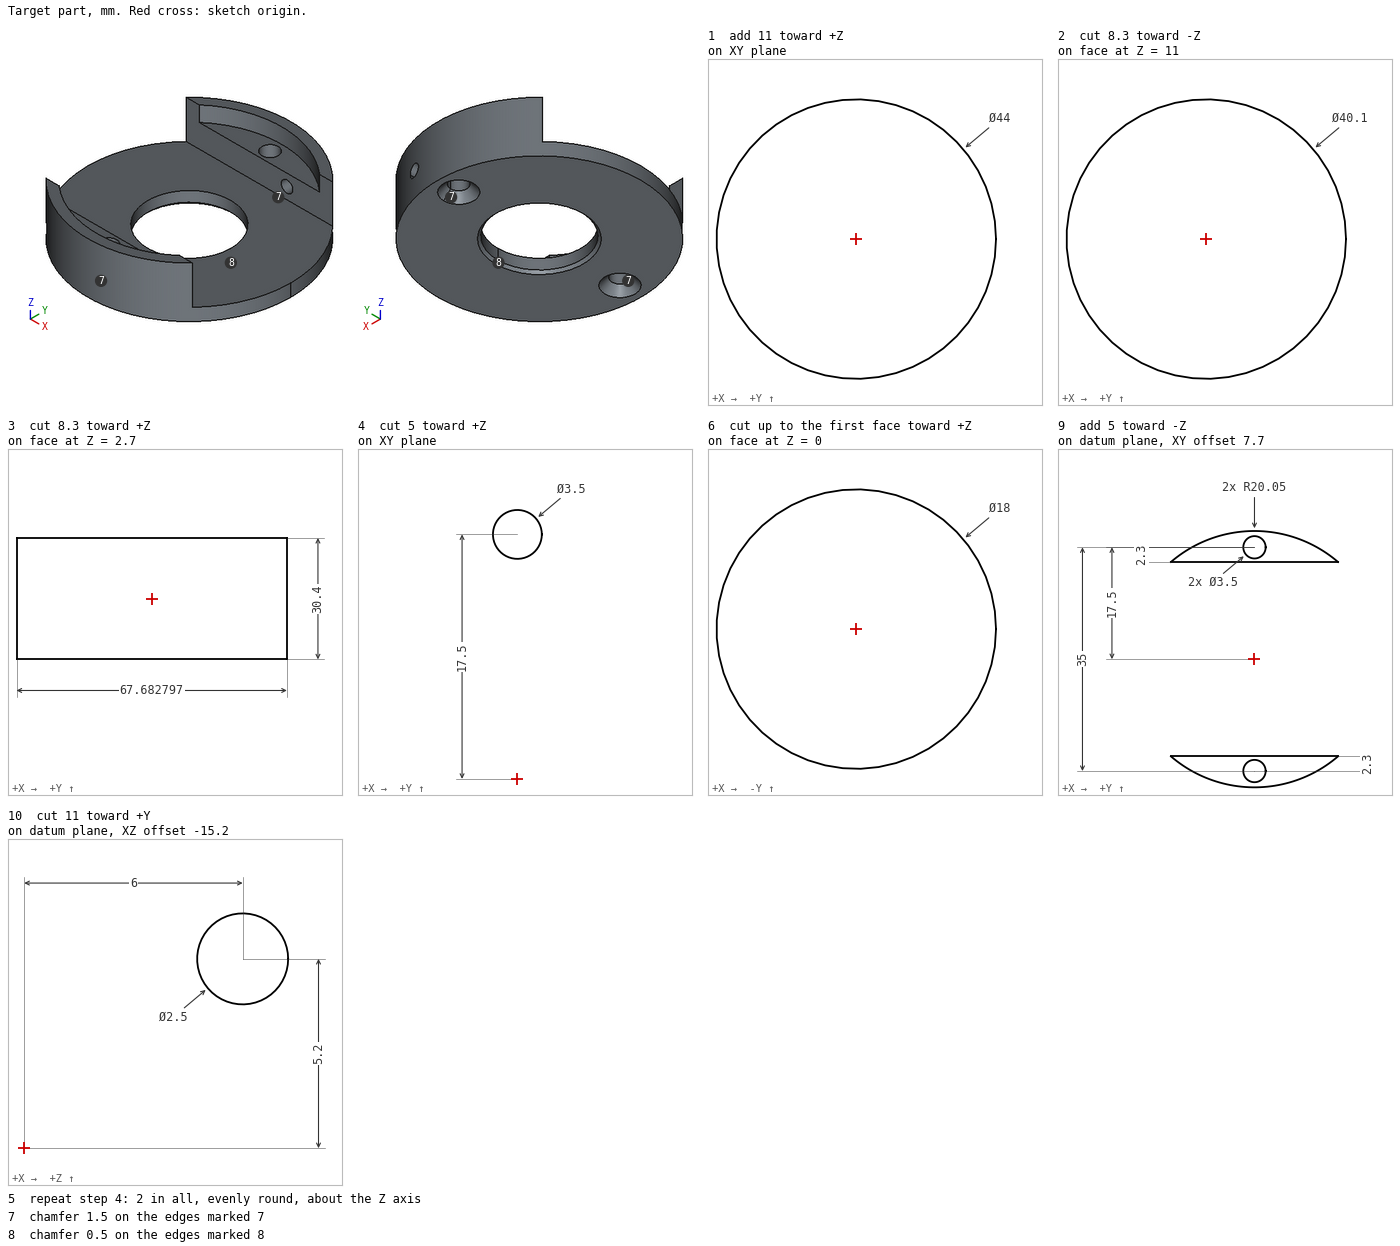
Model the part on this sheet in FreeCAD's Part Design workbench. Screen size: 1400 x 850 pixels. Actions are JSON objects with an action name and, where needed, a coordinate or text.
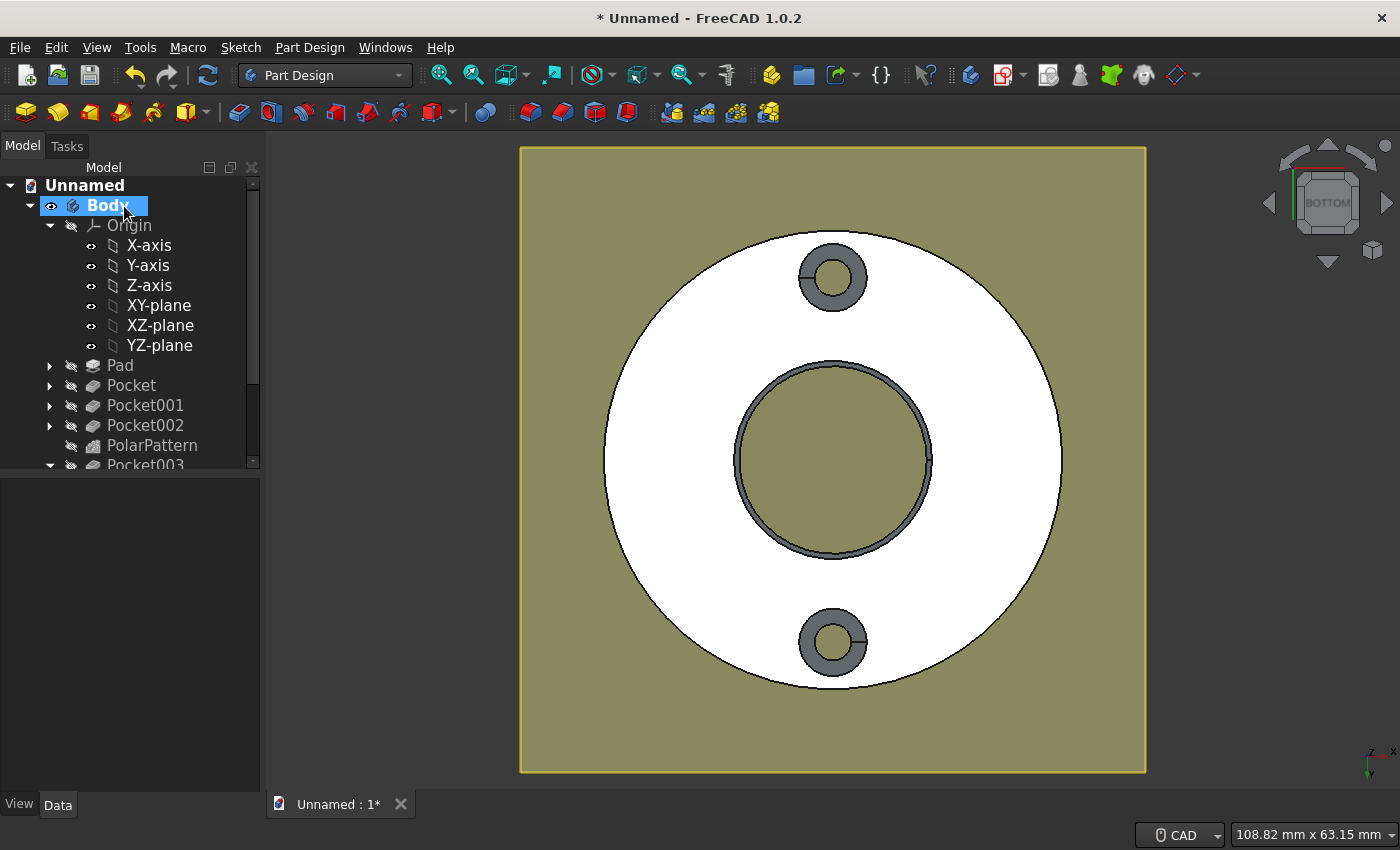
{"action": "scroll", "coordinate": [100, 321], "scroll_direction": "down", "scroll_amount": 3}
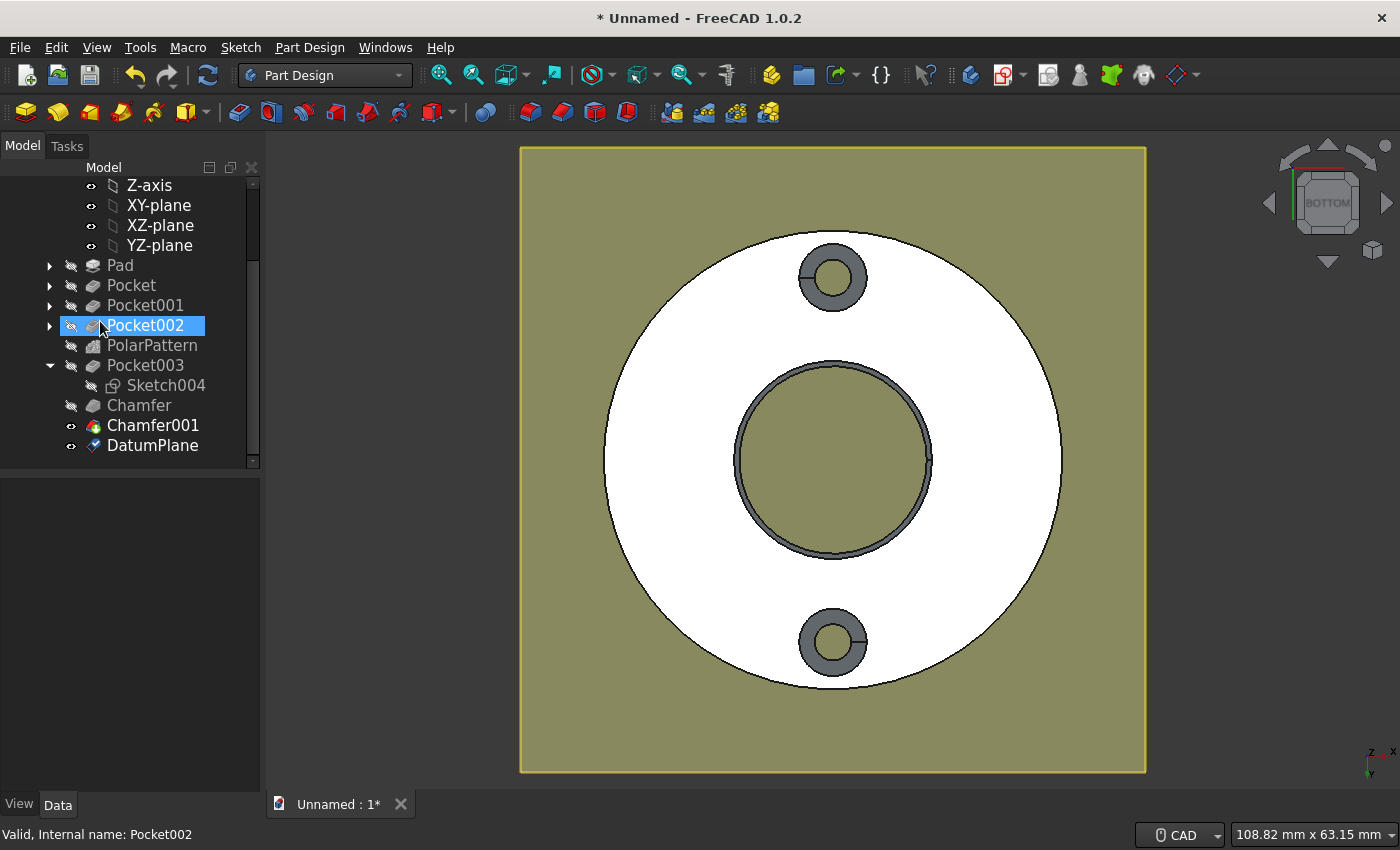
{"action": "left_click", "coordinate": [116, 446]}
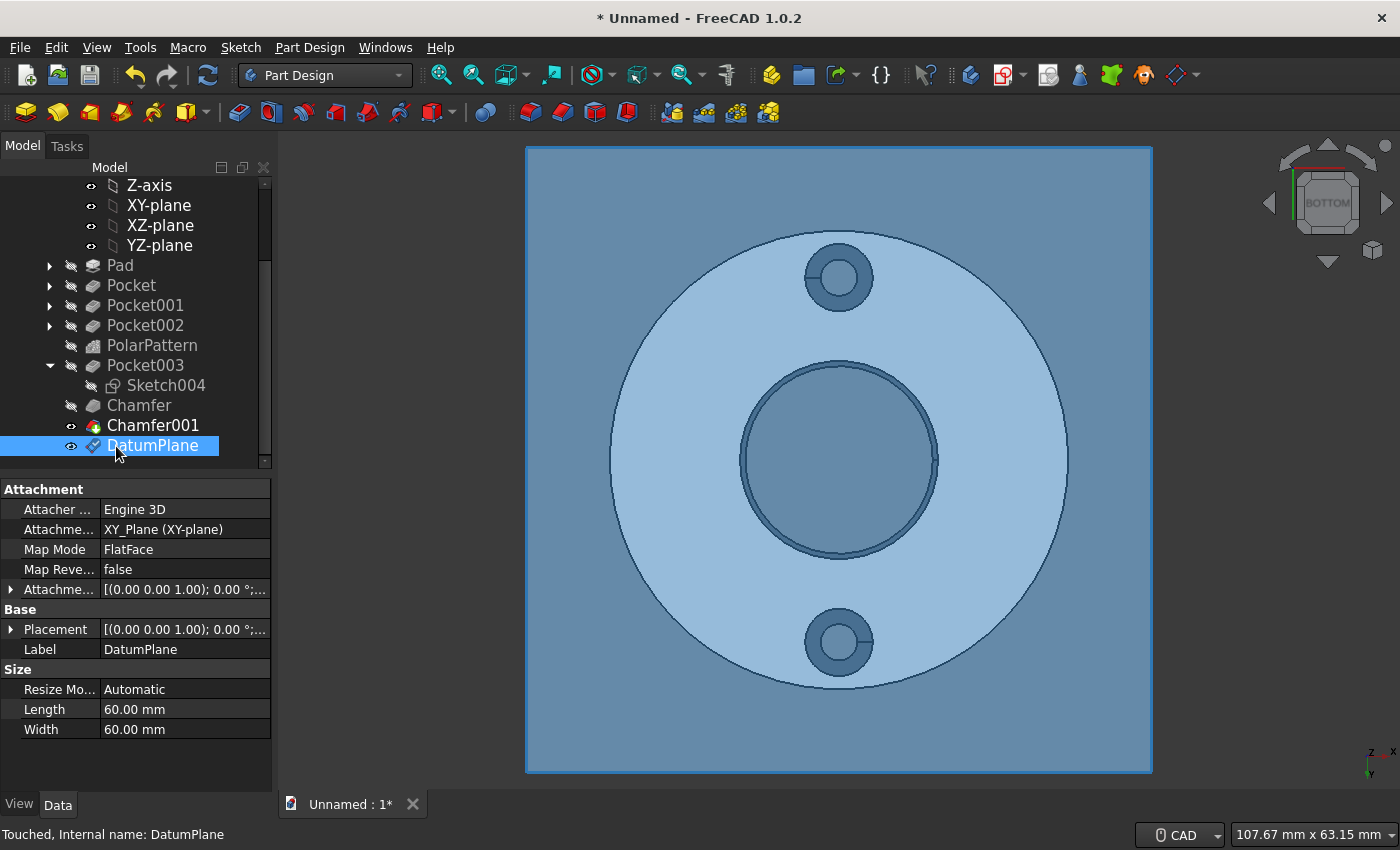
{"action": "left_click", "coordinate": [1004, 76]}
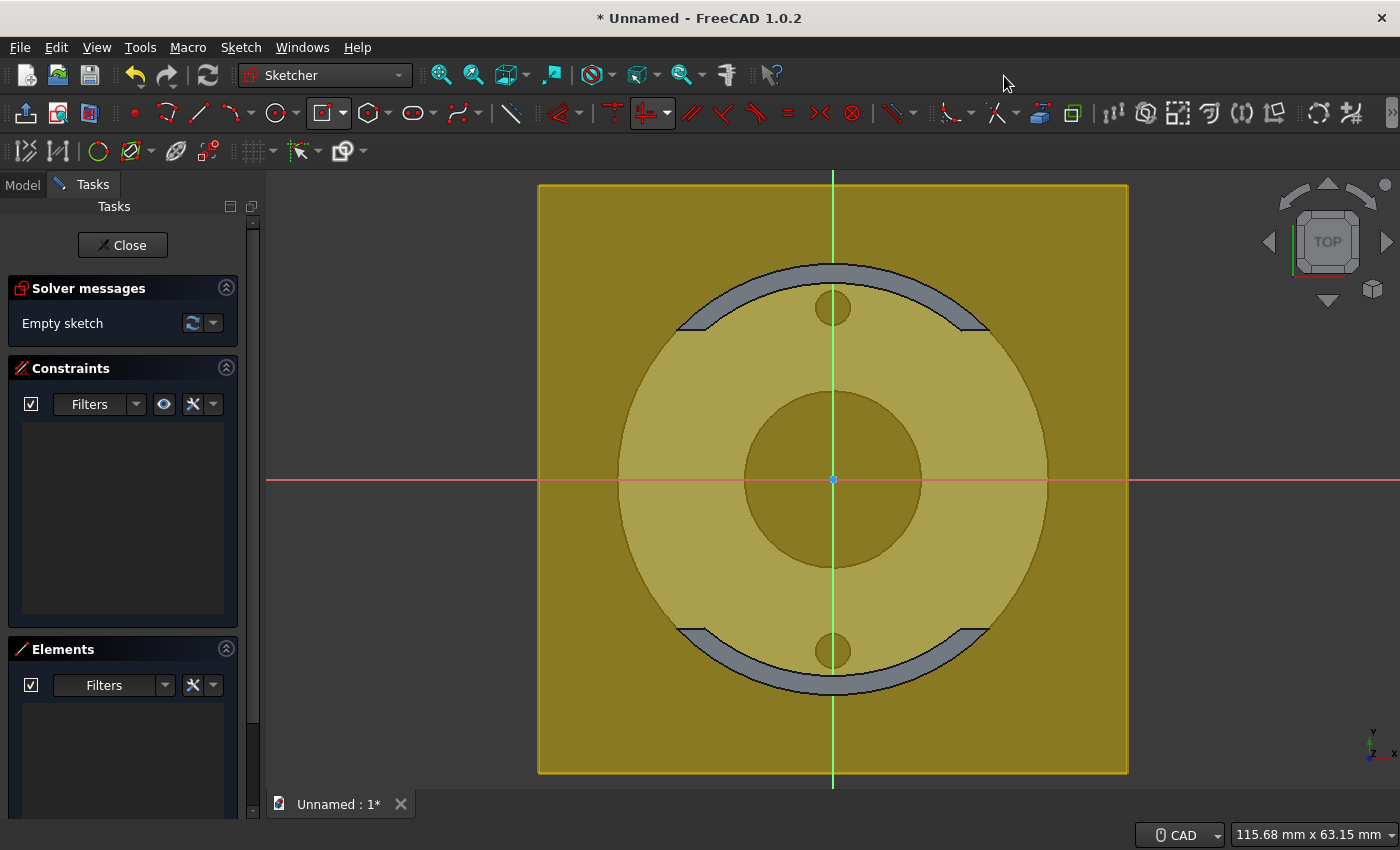
{"action": "left_click", "coordinate": [90, 114]}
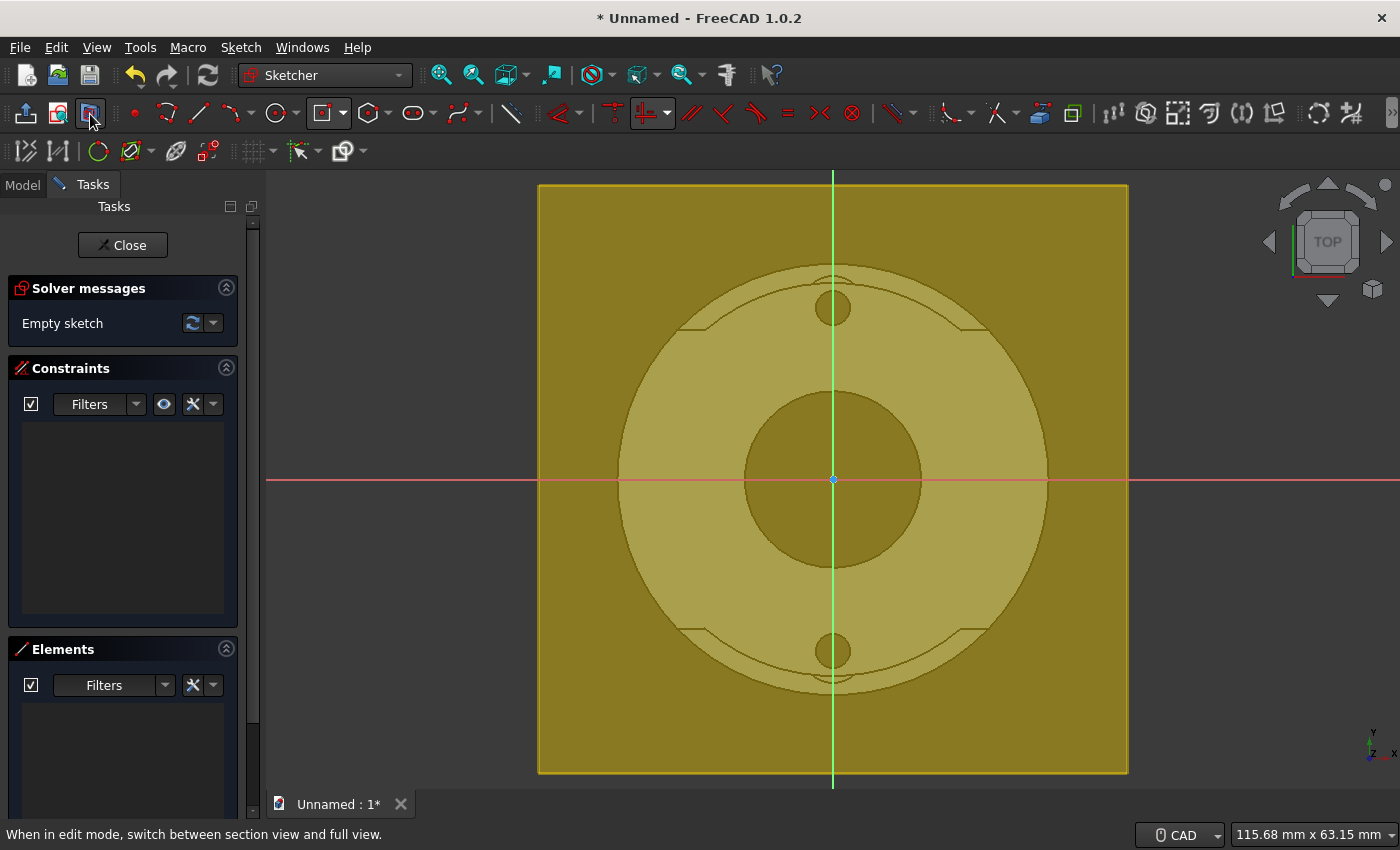
{"action": "key", "text": "g l"}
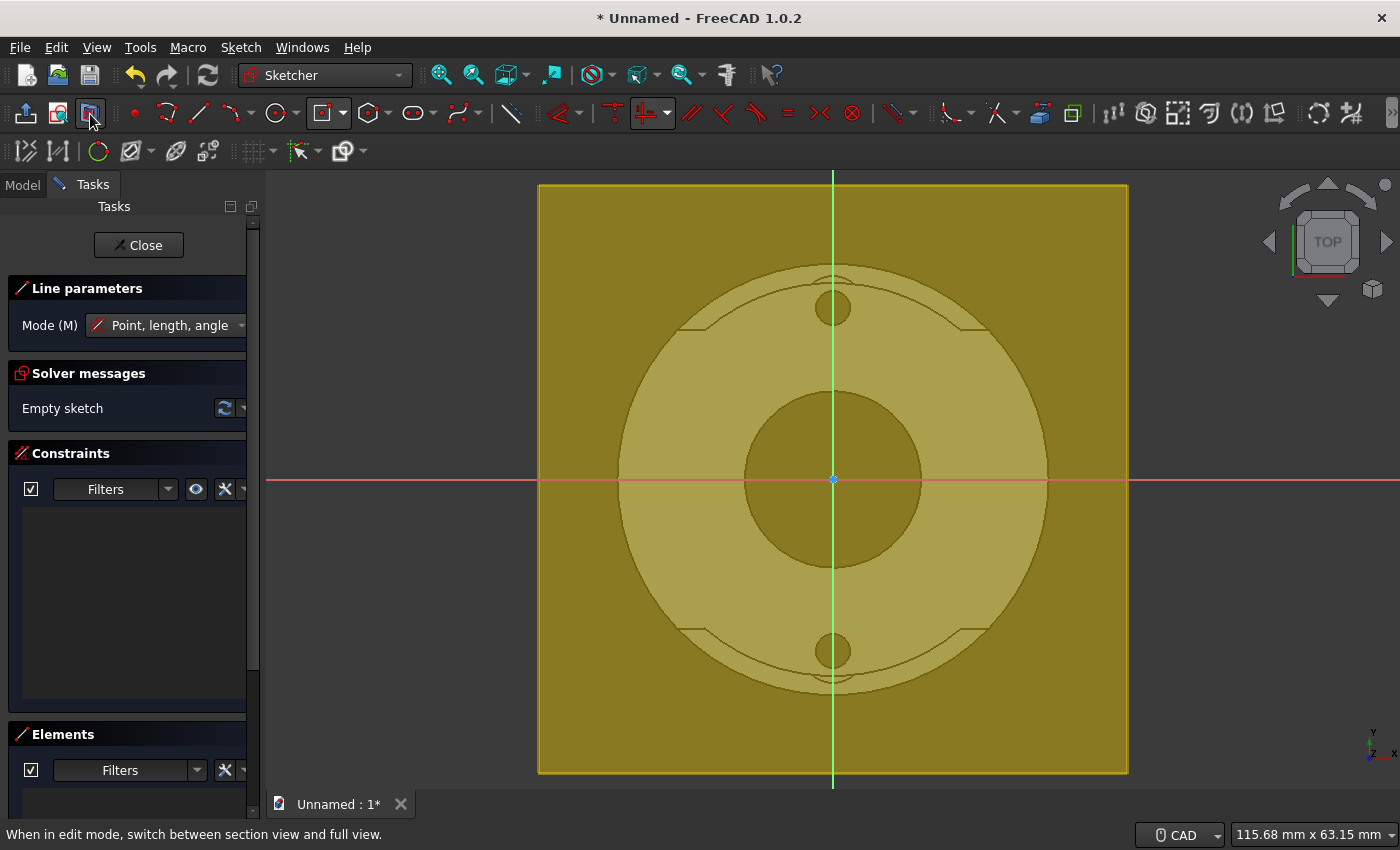
{"action": "left_click", "coordinate": [705, 330]}
{"action": "left_click", "coordinate": [961, 330]}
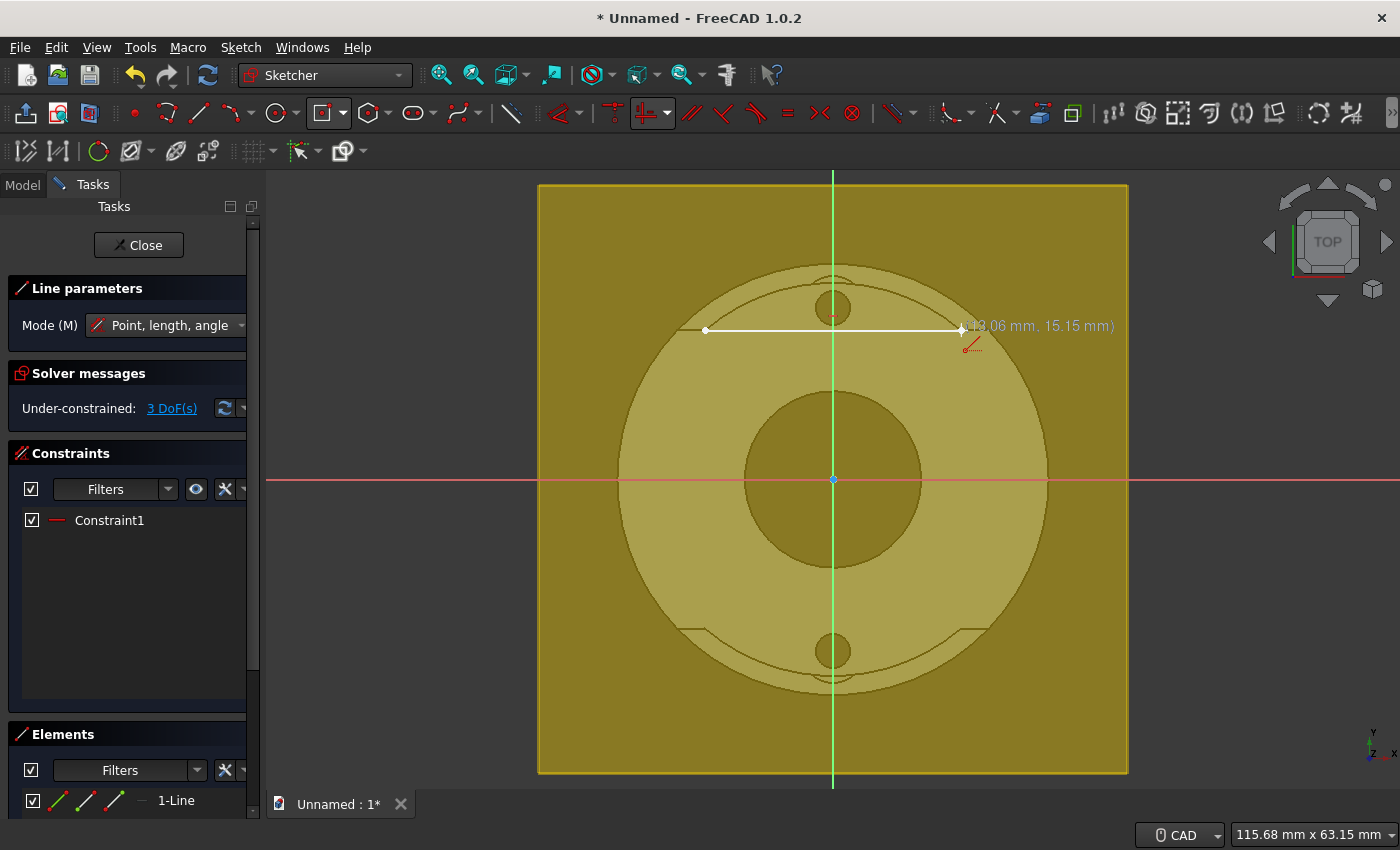
{"action": "key", "text": "g 3 a"}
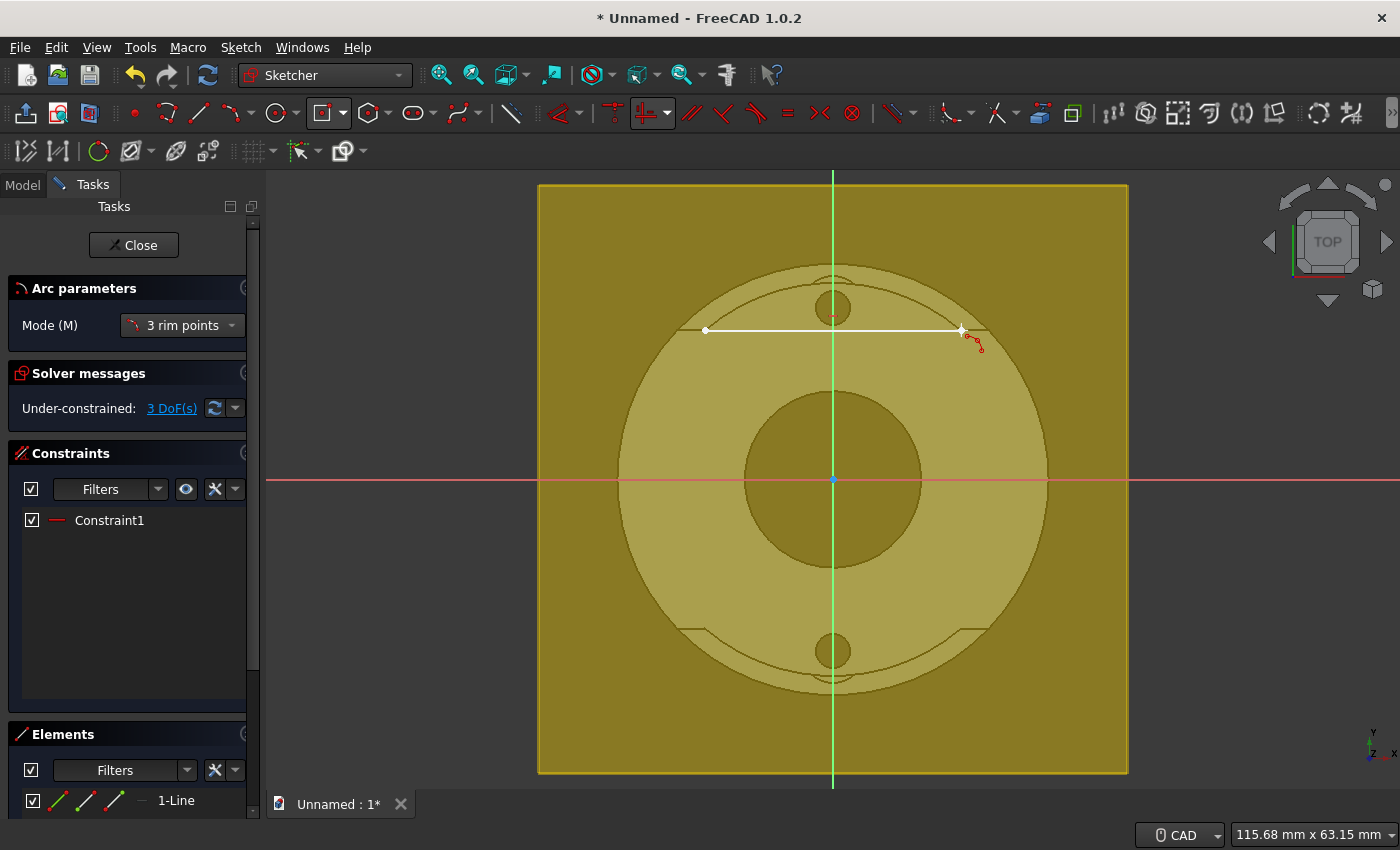
{"action": "left_click", "coordinate": [961, 331]}
{"action": "left_click", "coordinate": [705, 331]}
{"action": "left_click", "coordinate": [861, 285]}